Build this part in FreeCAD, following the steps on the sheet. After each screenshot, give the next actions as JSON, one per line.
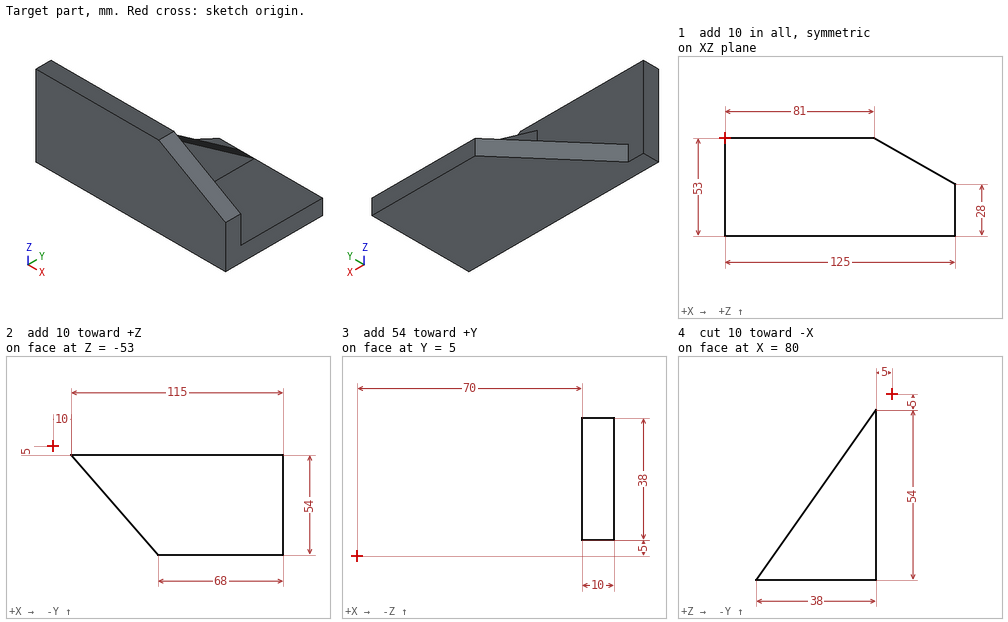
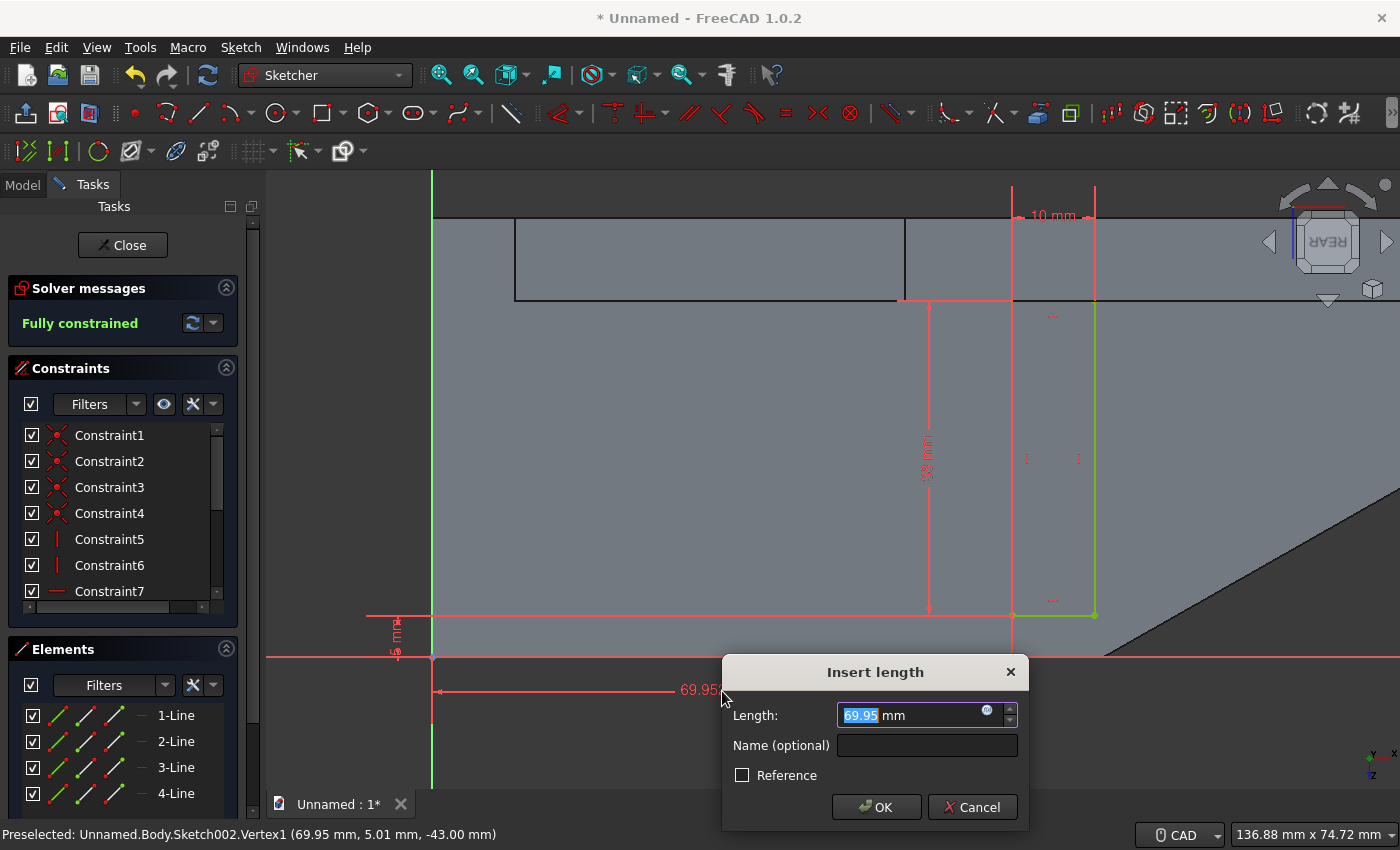
{"action": "type", "text": "70"}
{"action": "key", "text": "Return"}
{"action": "key", "text": "Escape"}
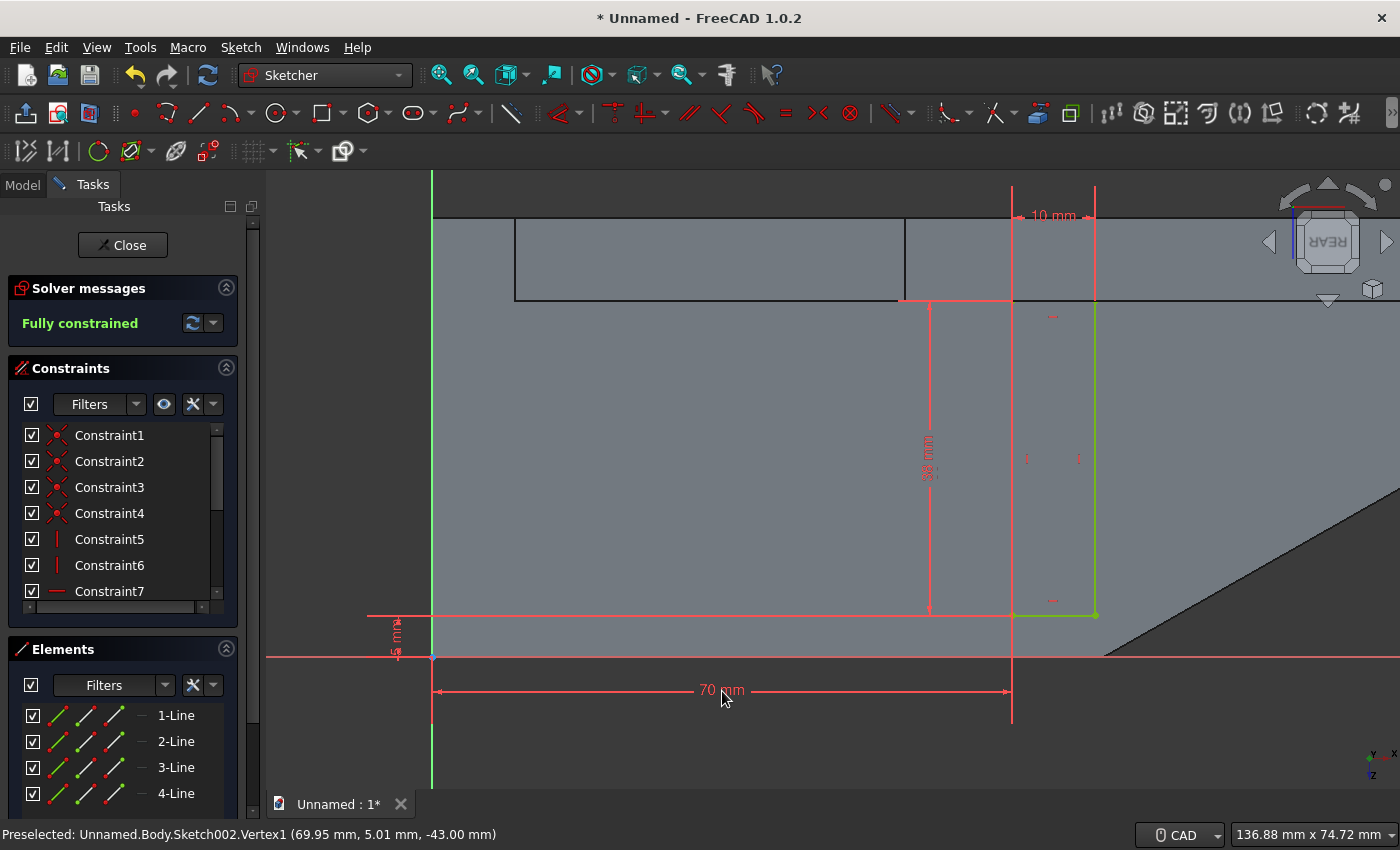
{"action": "left_click", "coordinate": [123, 245]}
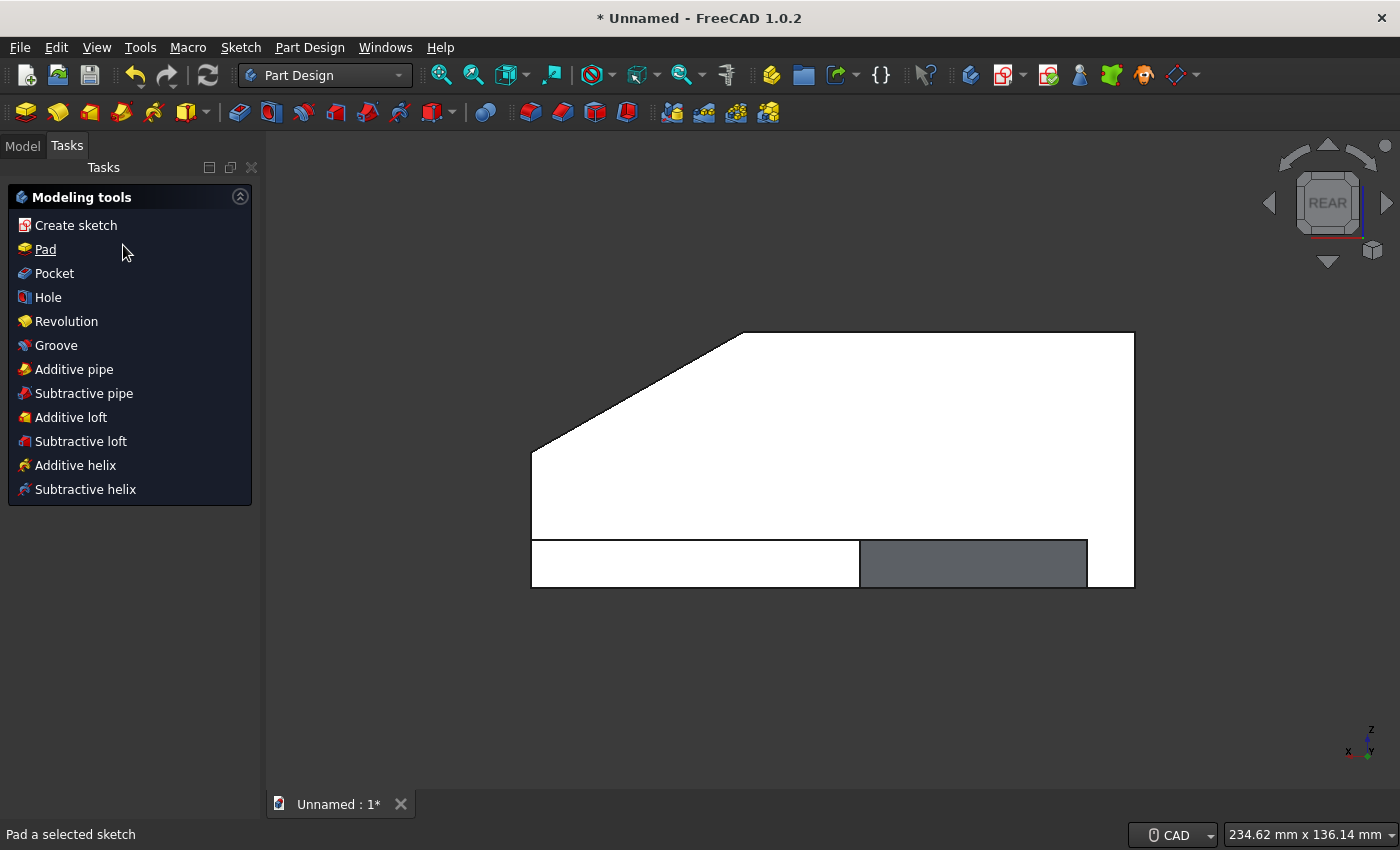
{"action": "left_click", "coordinate": [26, 112]}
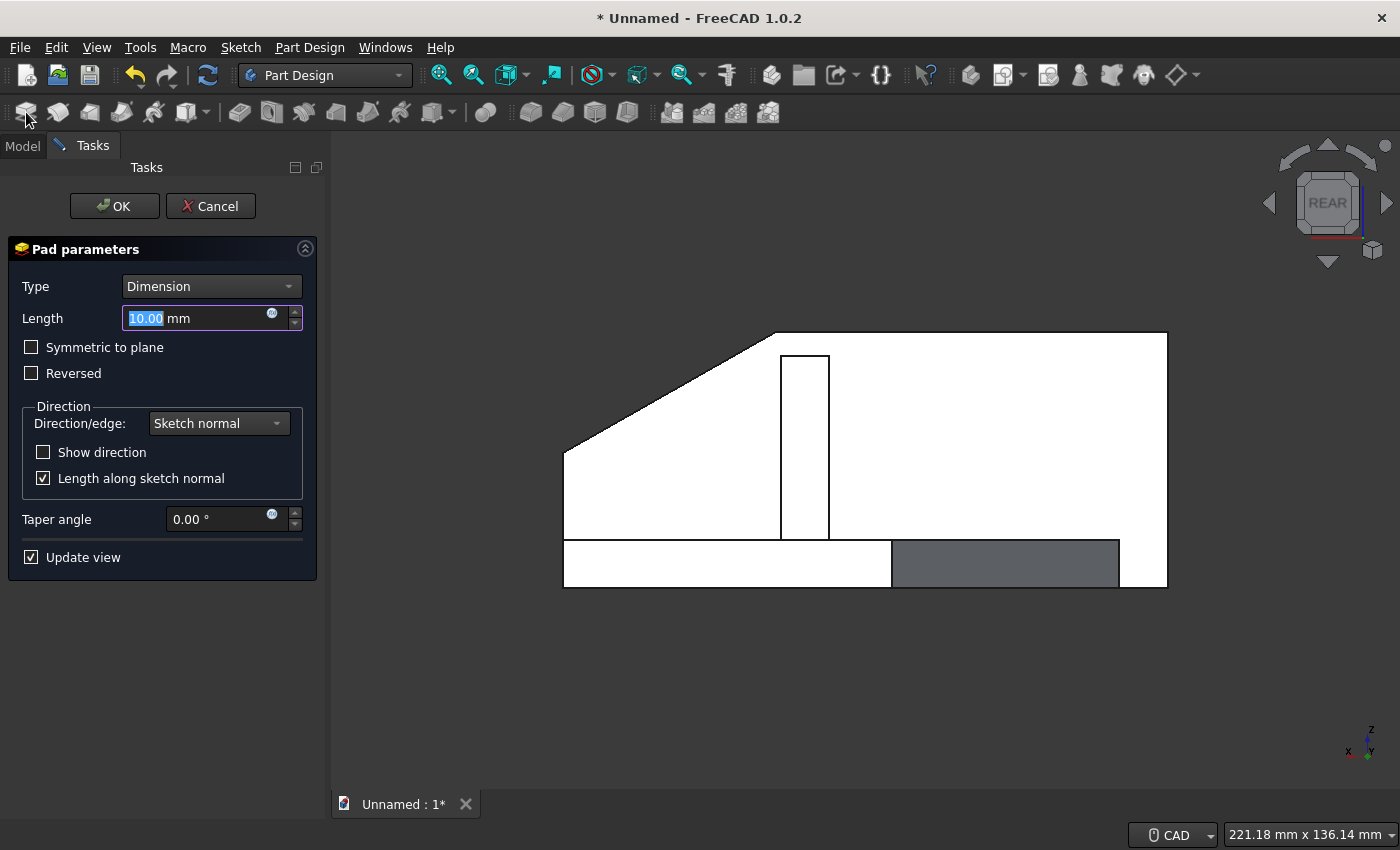
{"action": "type", "text": "54"}
{"action": "key", "text": "Tab"}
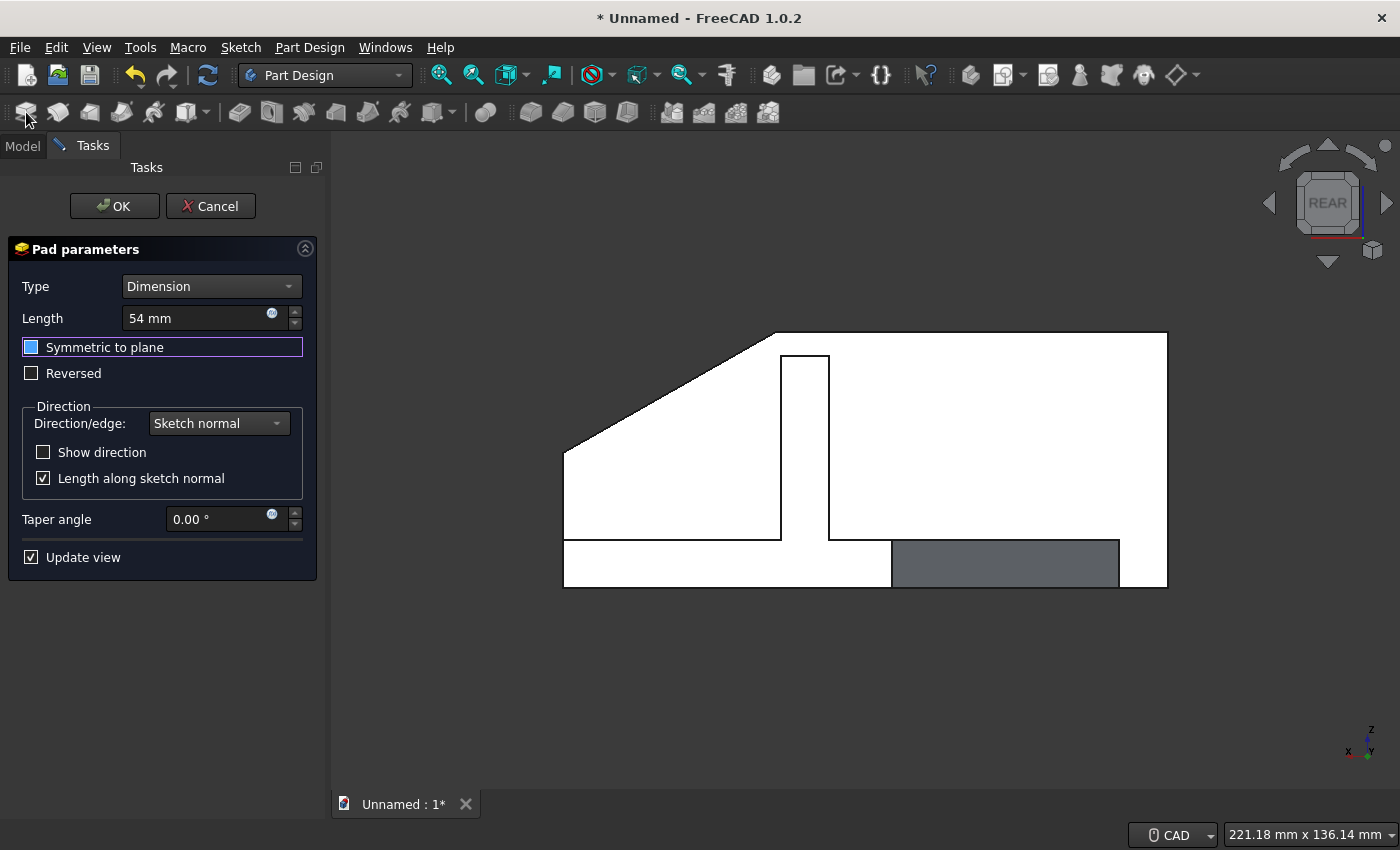
{"action": "left_click", "coordinate": [115, 206]}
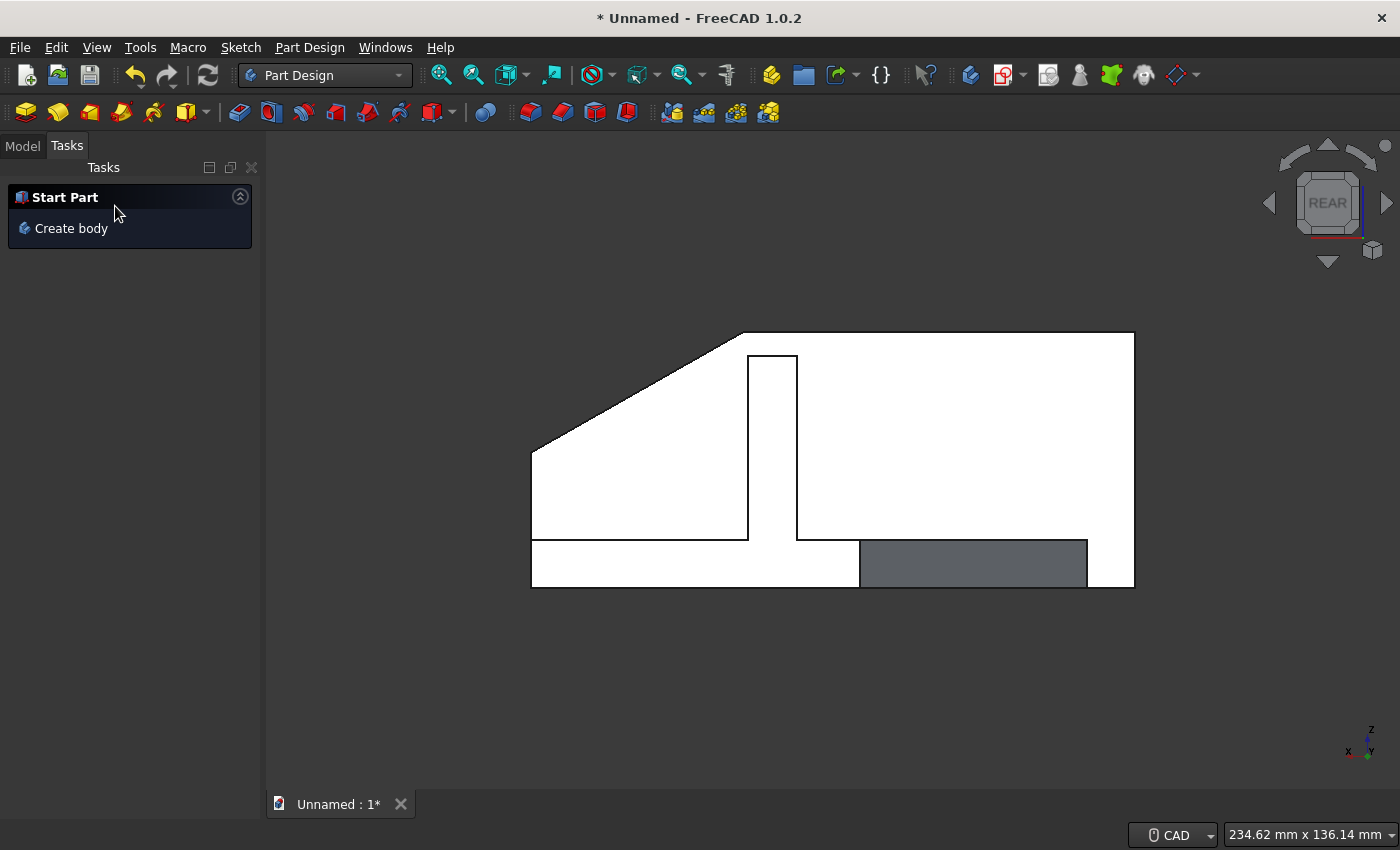
{"action": "key", "text": "0"}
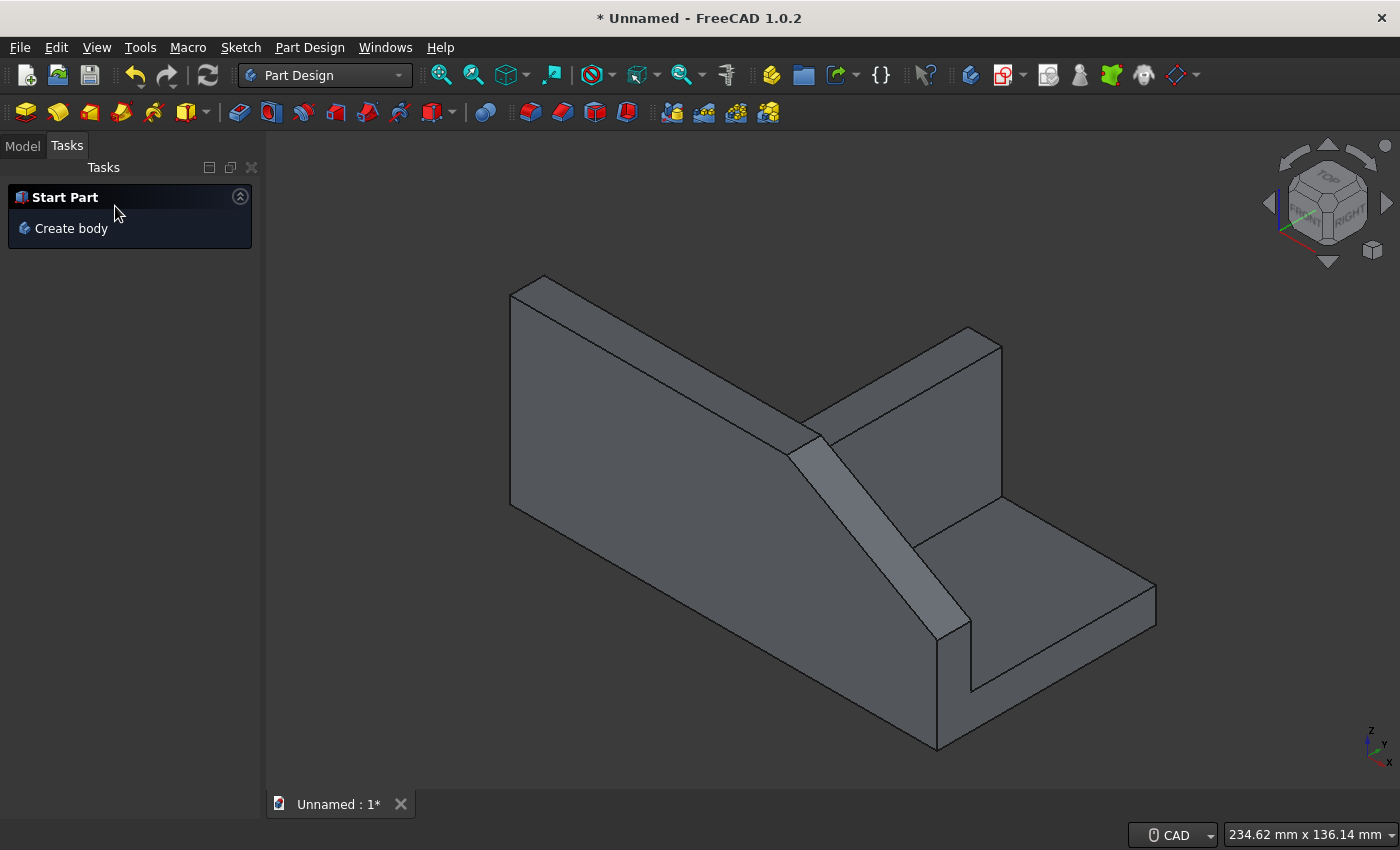
{"action": "left_click", "coordinate": [936, 459]}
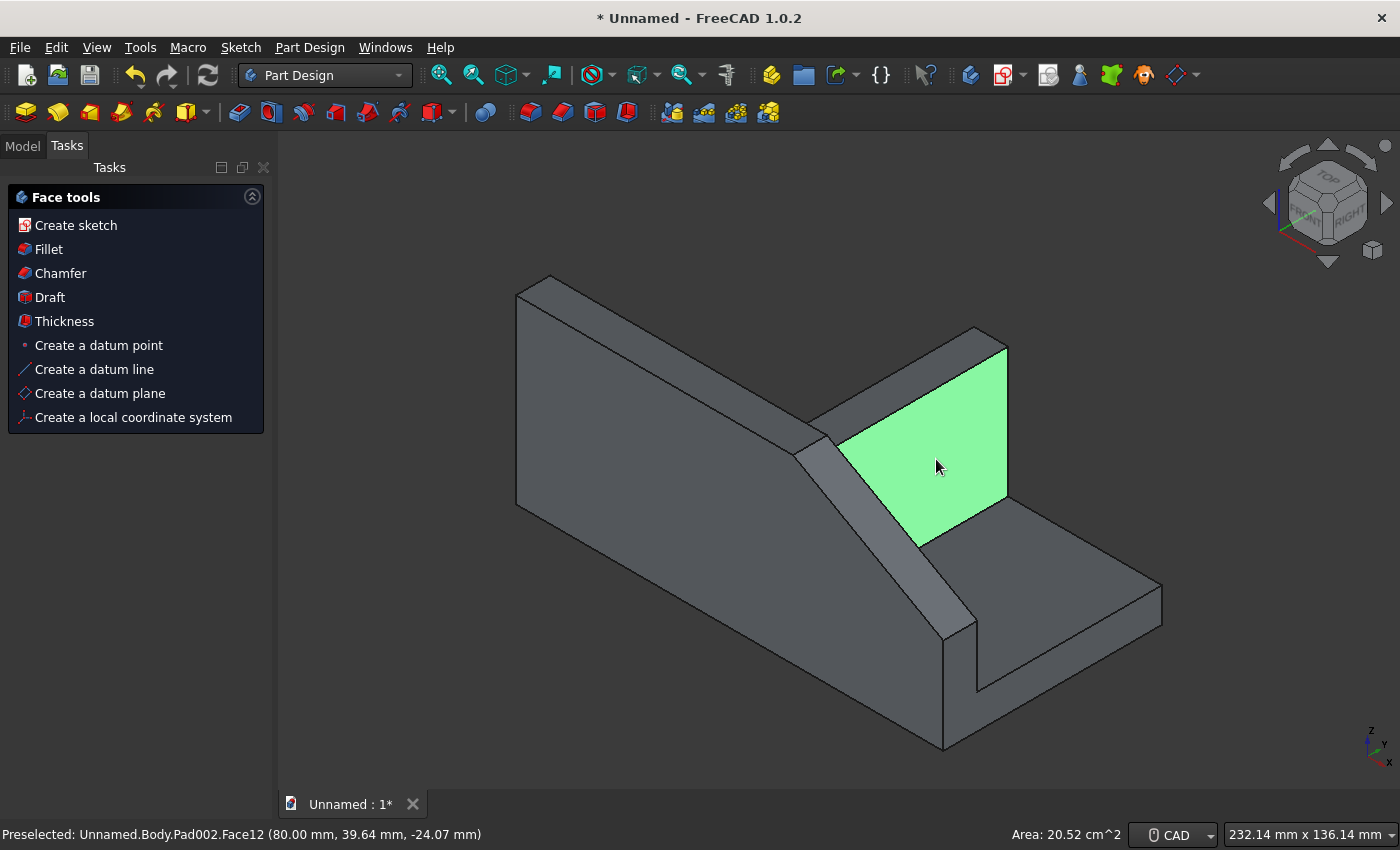
{"action": "left_click", "coordinate": [1004, 76]}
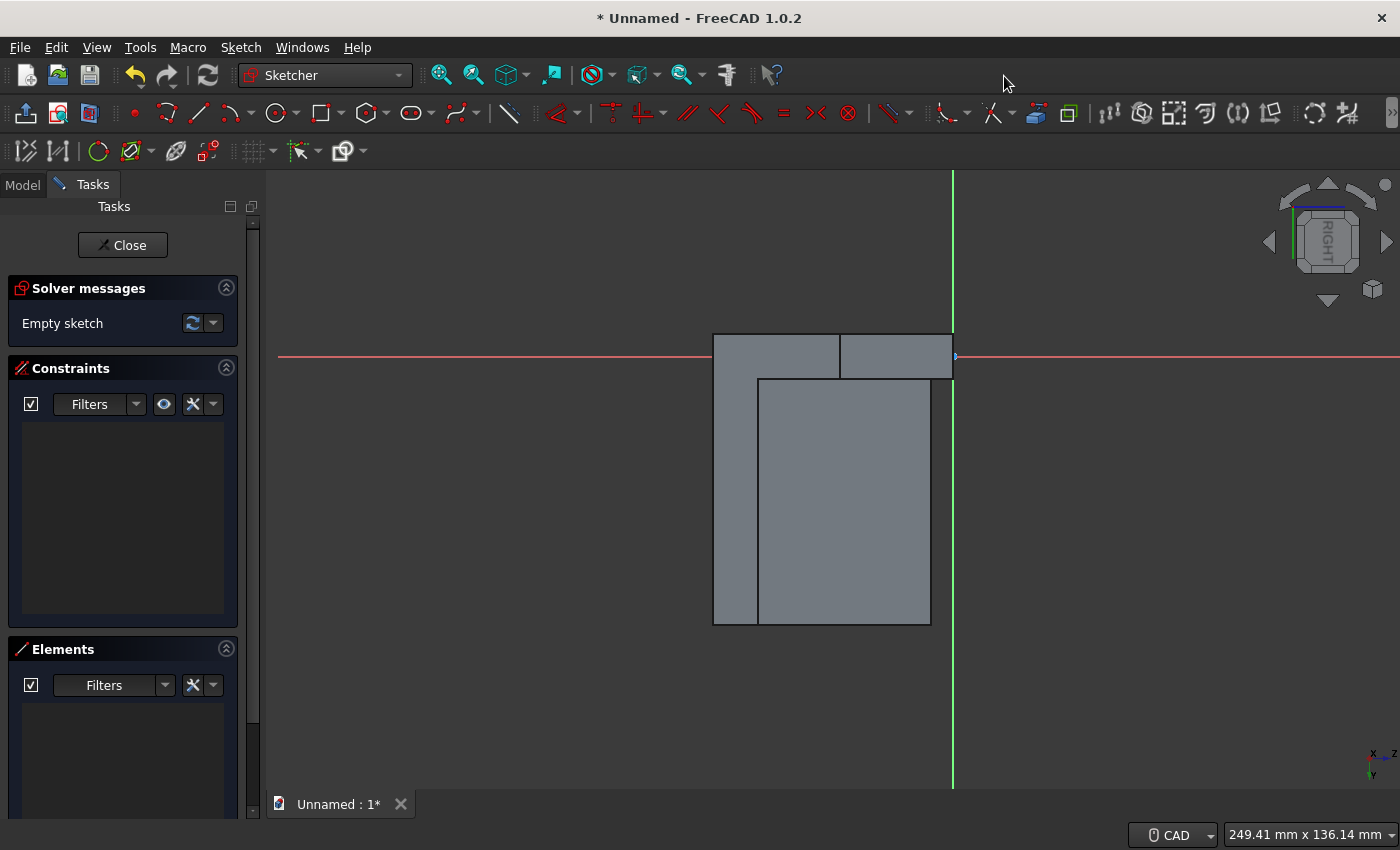
{"action": "key", "text": "q s"}